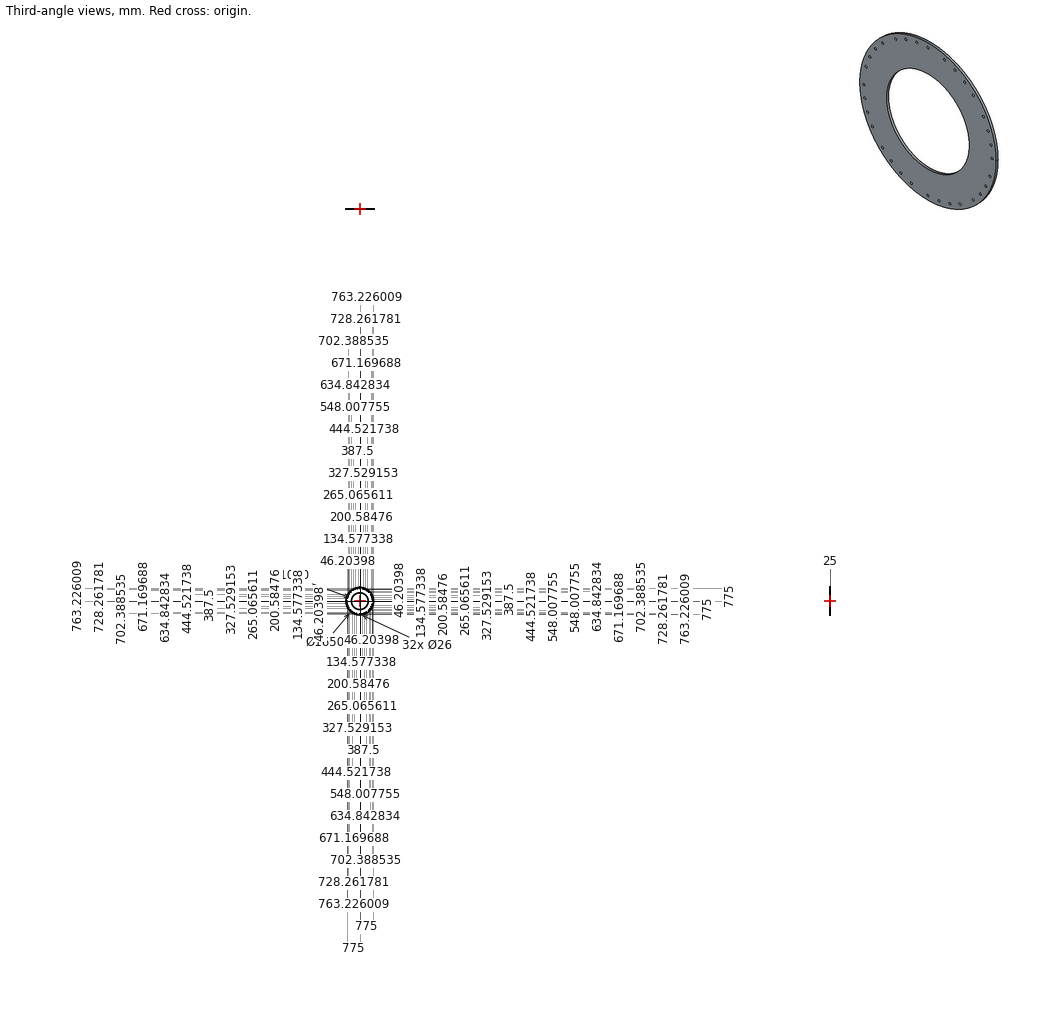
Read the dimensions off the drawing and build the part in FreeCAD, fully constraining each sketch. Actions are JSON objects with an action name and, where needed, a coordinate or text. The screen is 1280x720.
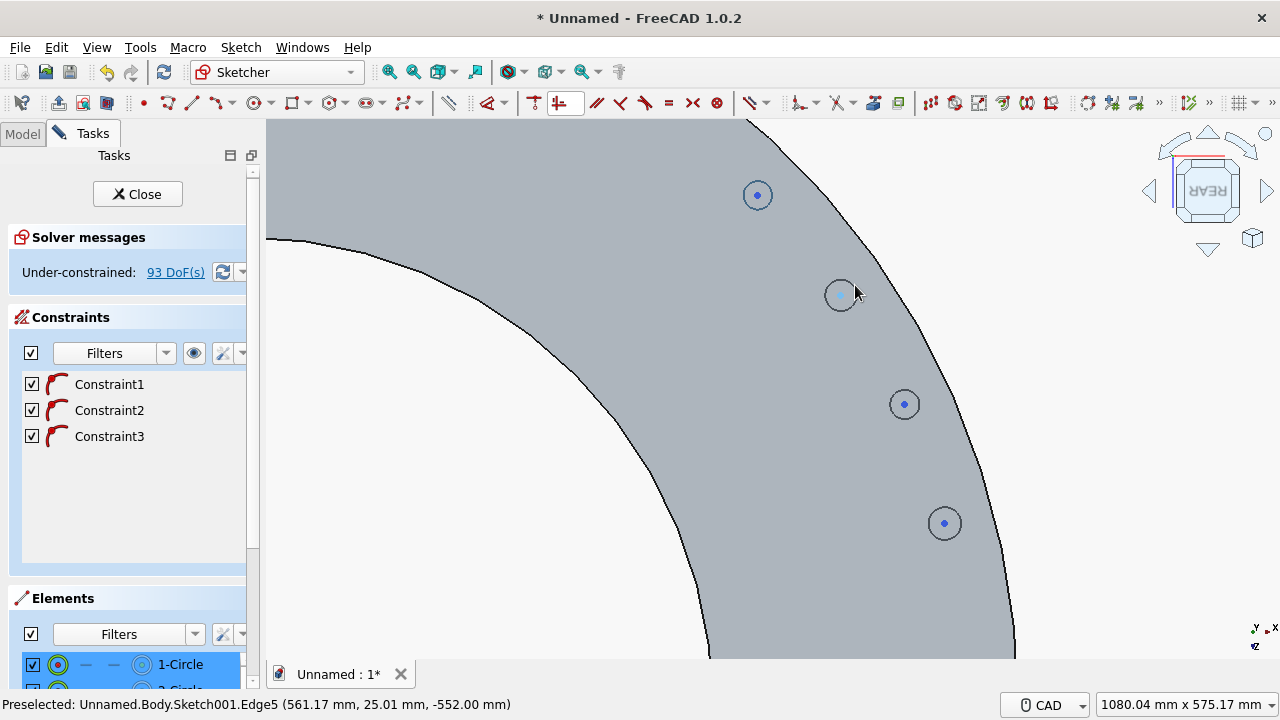
{"action": "left_click", "coordinate": [852, 284]}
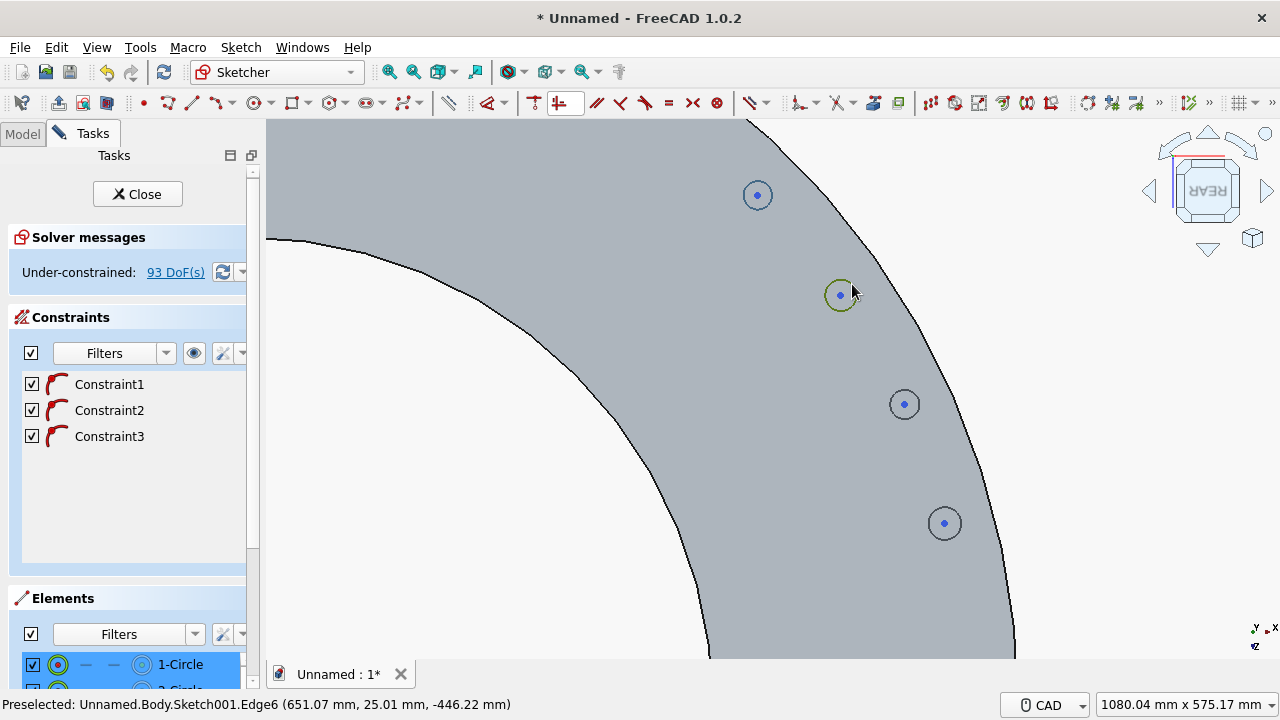
{"action": "left_click", "coordinate": [915, 394]}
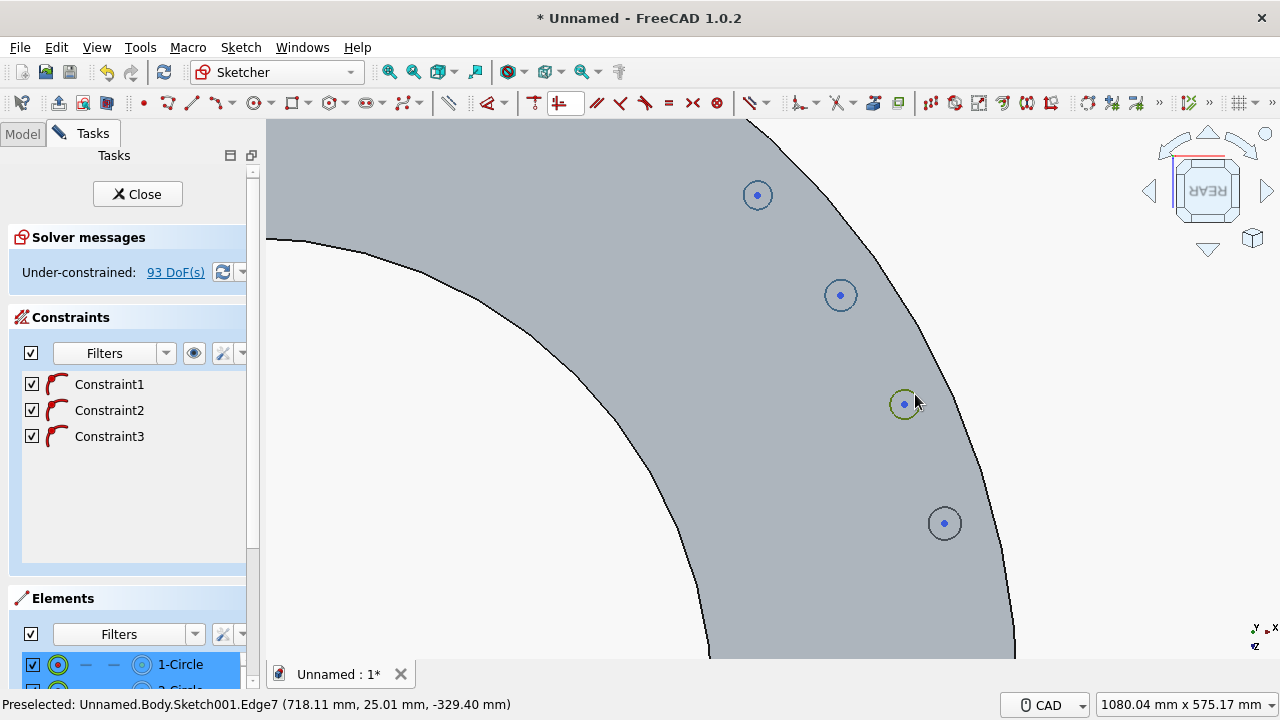
{"action": "left_click", "coordinate": [956, 512]}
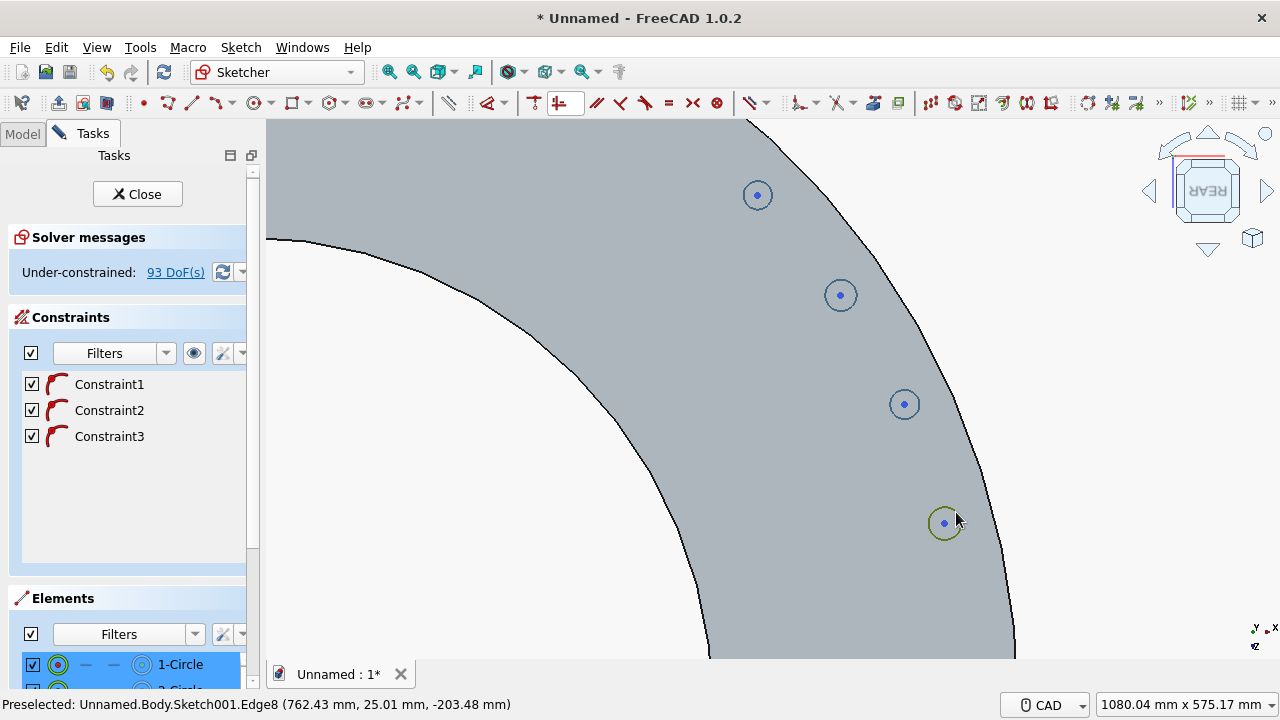
{"action": "scroll", "coordinate": [855, 285], "scroll_direction": "down", "scroll_amount": 7}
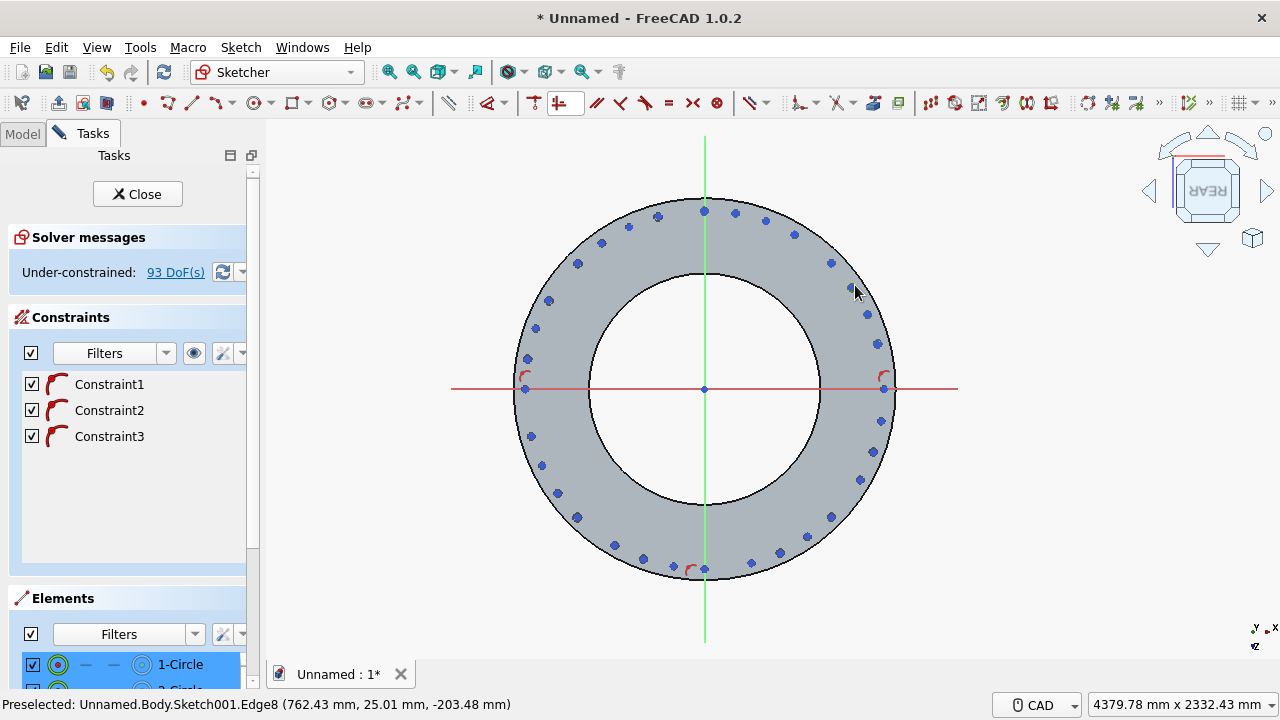
{"action": "scroll", "coordinate": [886, 387], "scroll_direction": "up", "scroll_amount": 10}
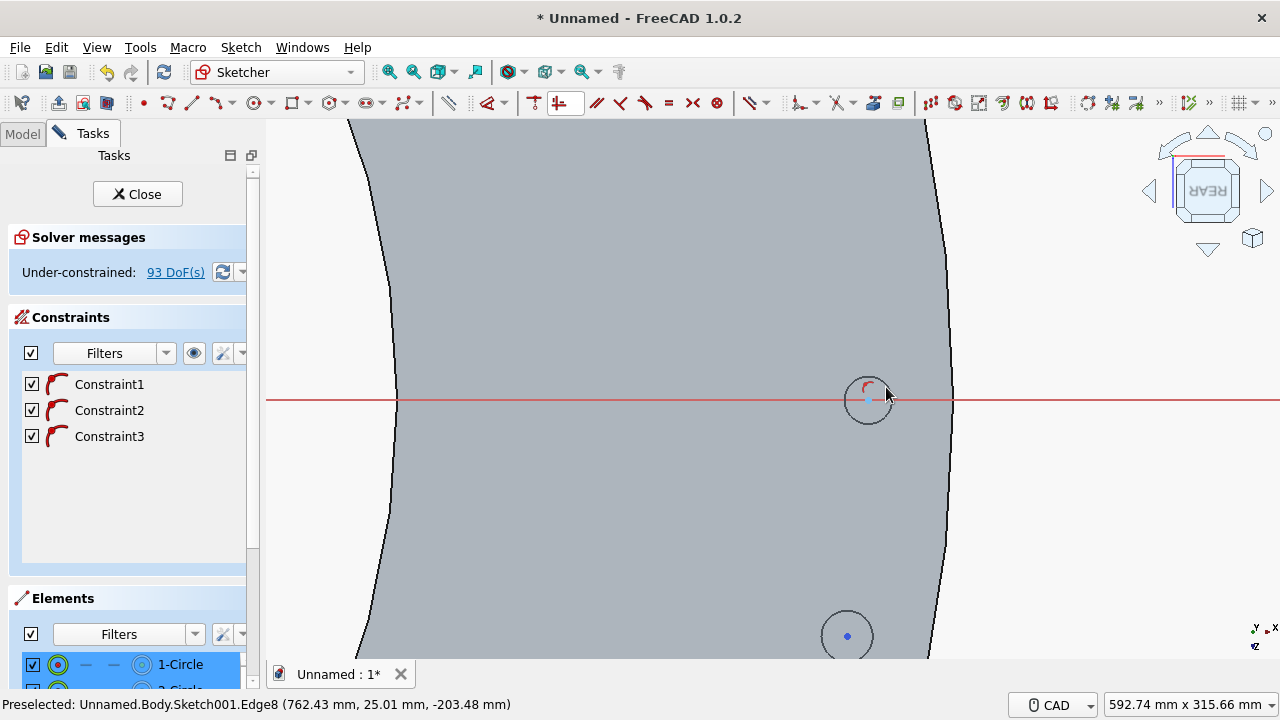
{"action": "left_click", "coordinate": [885, 383]}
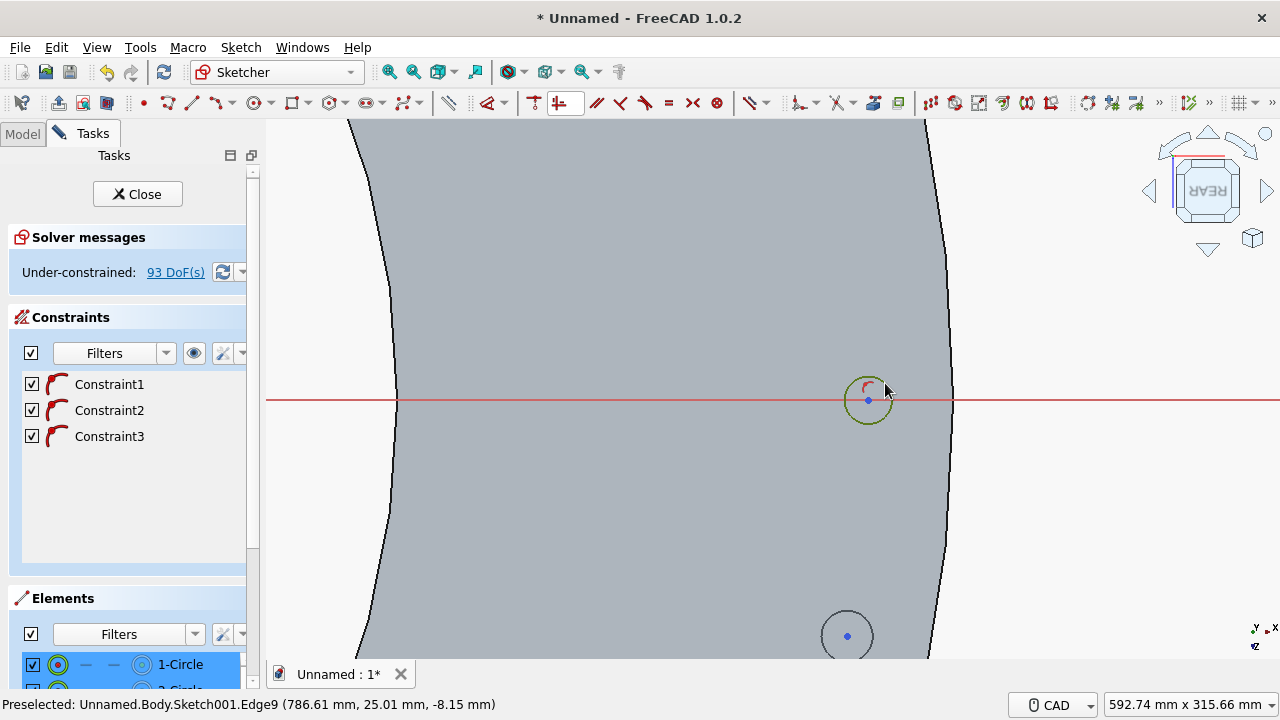
{"action": "left_click", "coordinate": [865, 618]}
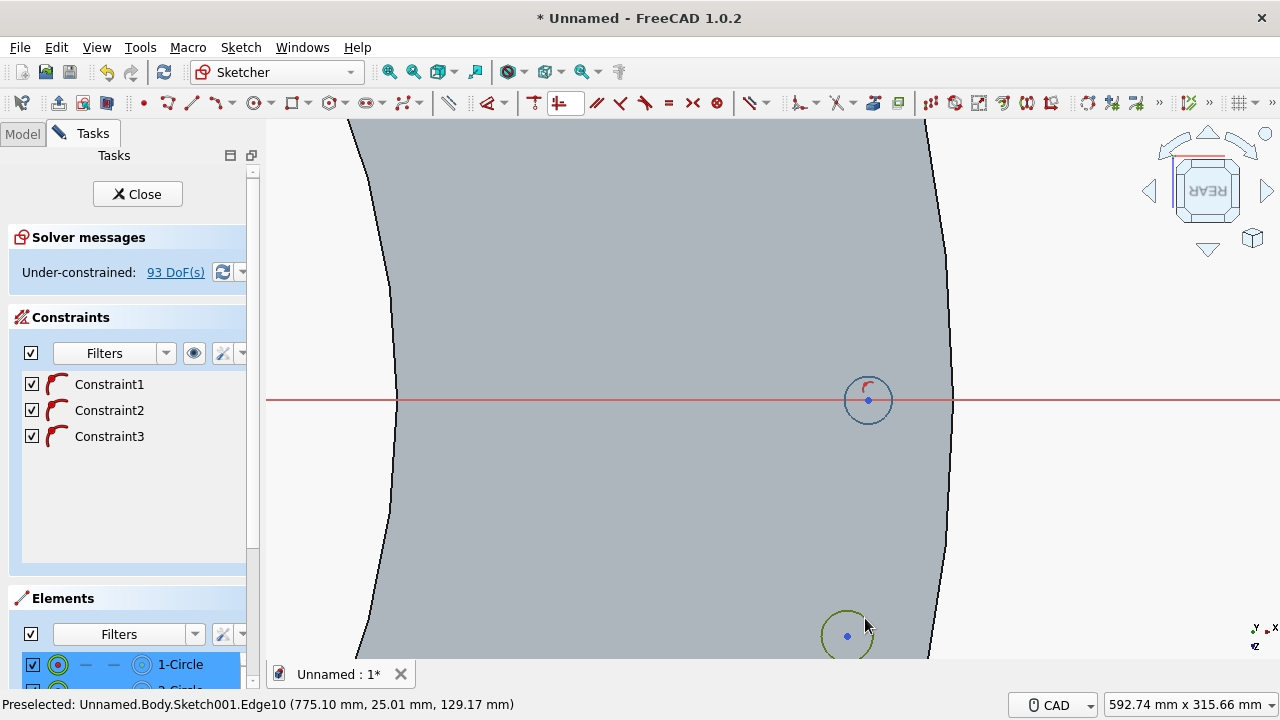
{"action": "scroll", "coordinate": [886, 387], "scroll_direction": "down", "scroll_amount": 10}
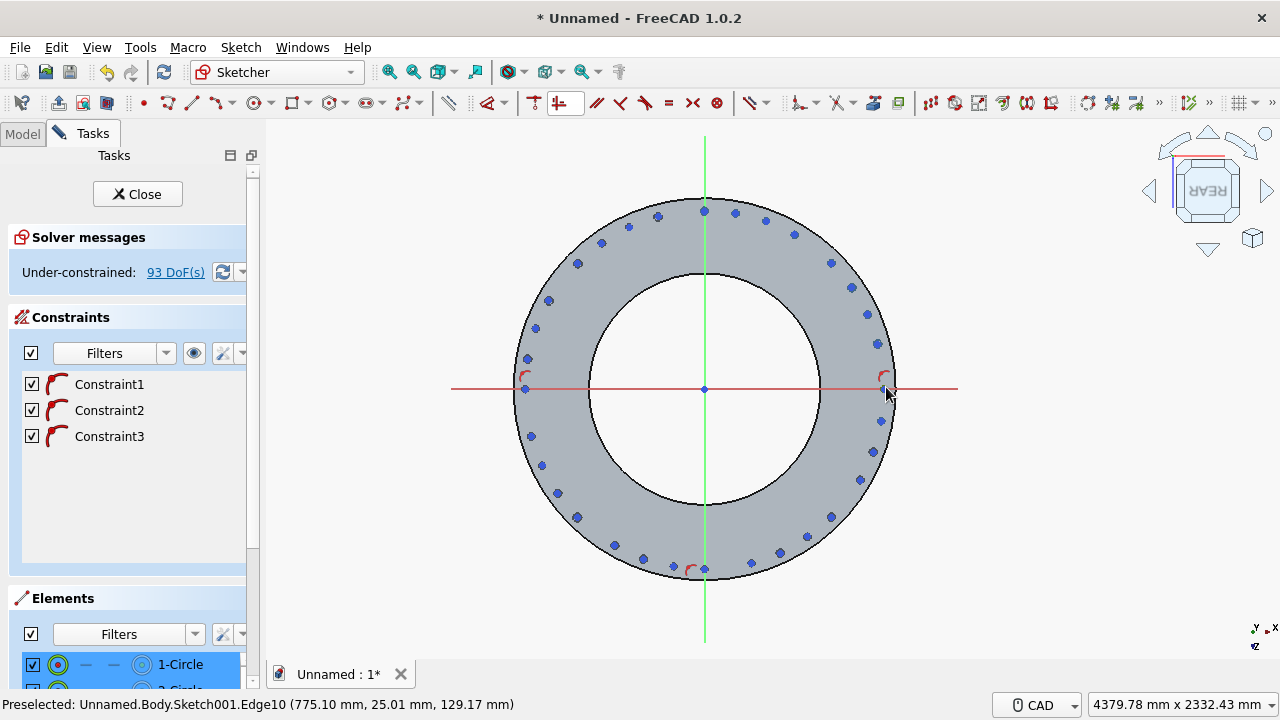
{"action": "scroll", "coordinate": [876, 449], "scroll_direction": "up", "scroll_amount": 7}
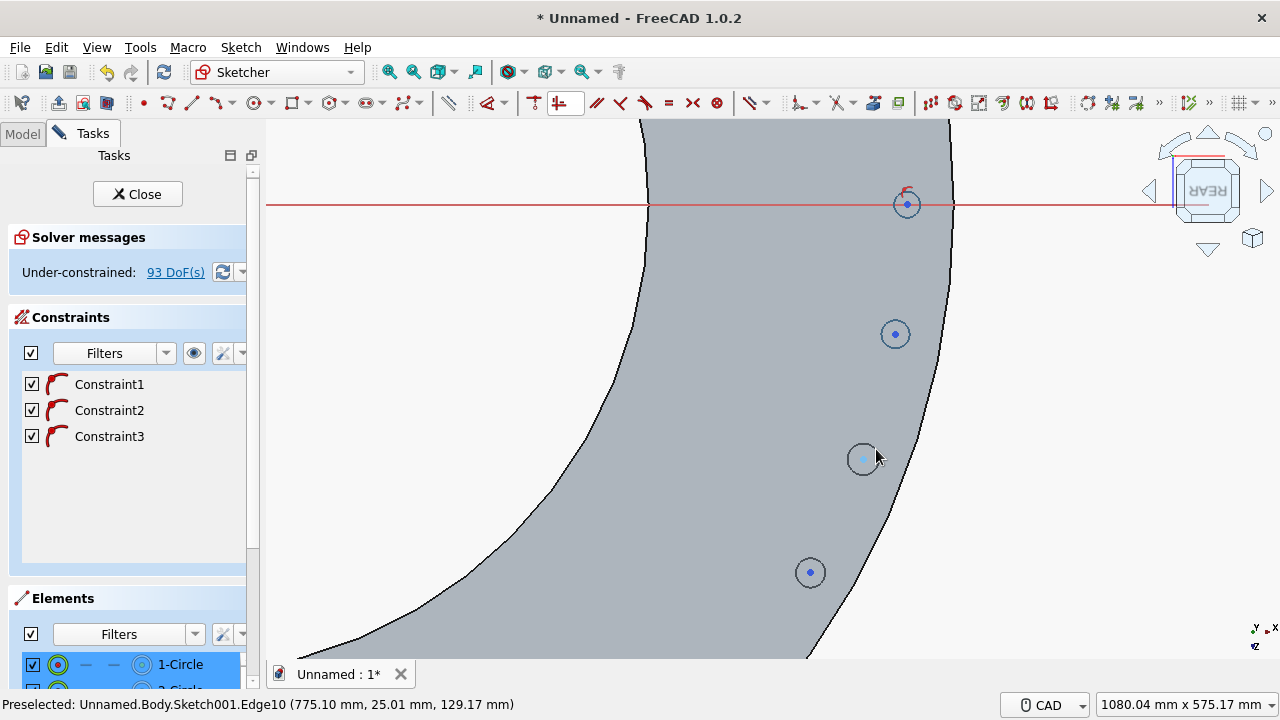
{"action": "left_click", "coordinate": [874, 448]}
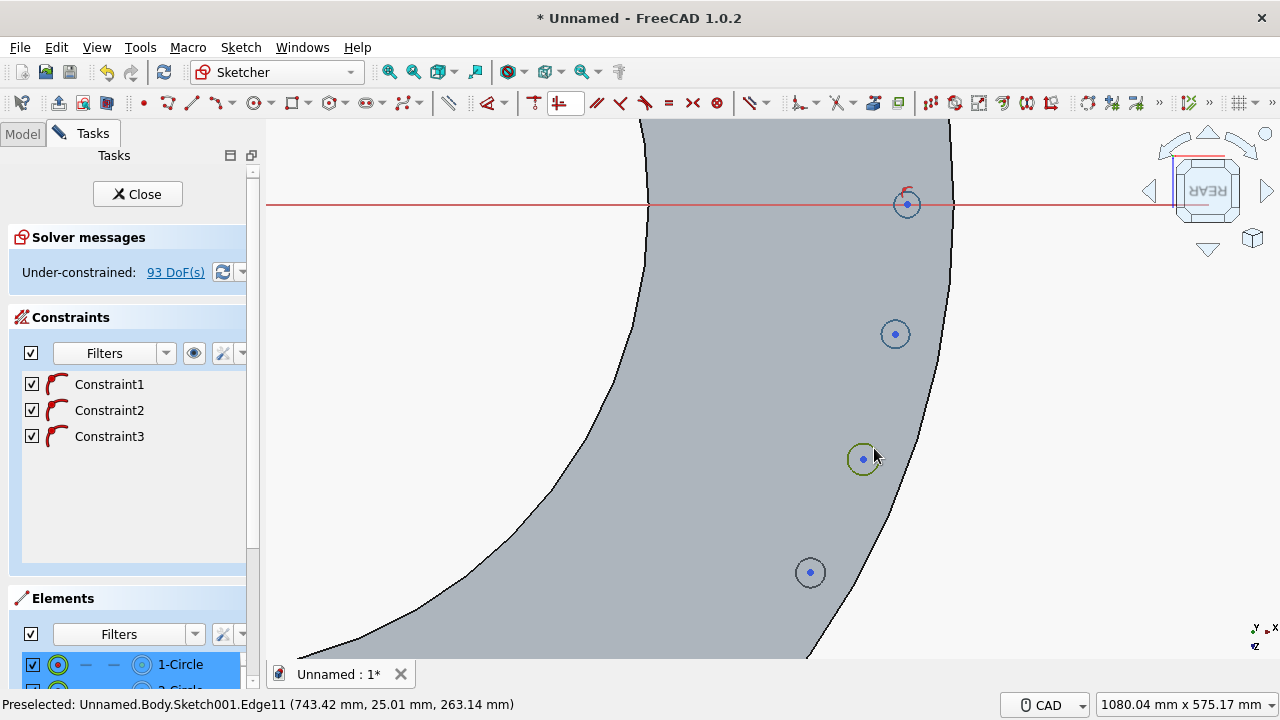
{"action": "left_click", "coordinate": [821, 563]}